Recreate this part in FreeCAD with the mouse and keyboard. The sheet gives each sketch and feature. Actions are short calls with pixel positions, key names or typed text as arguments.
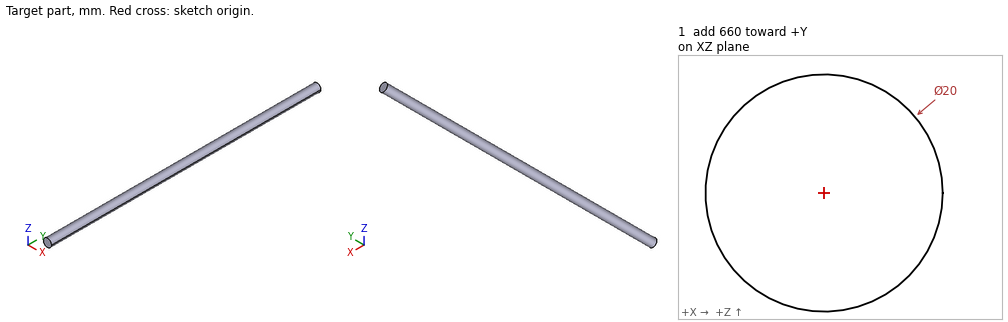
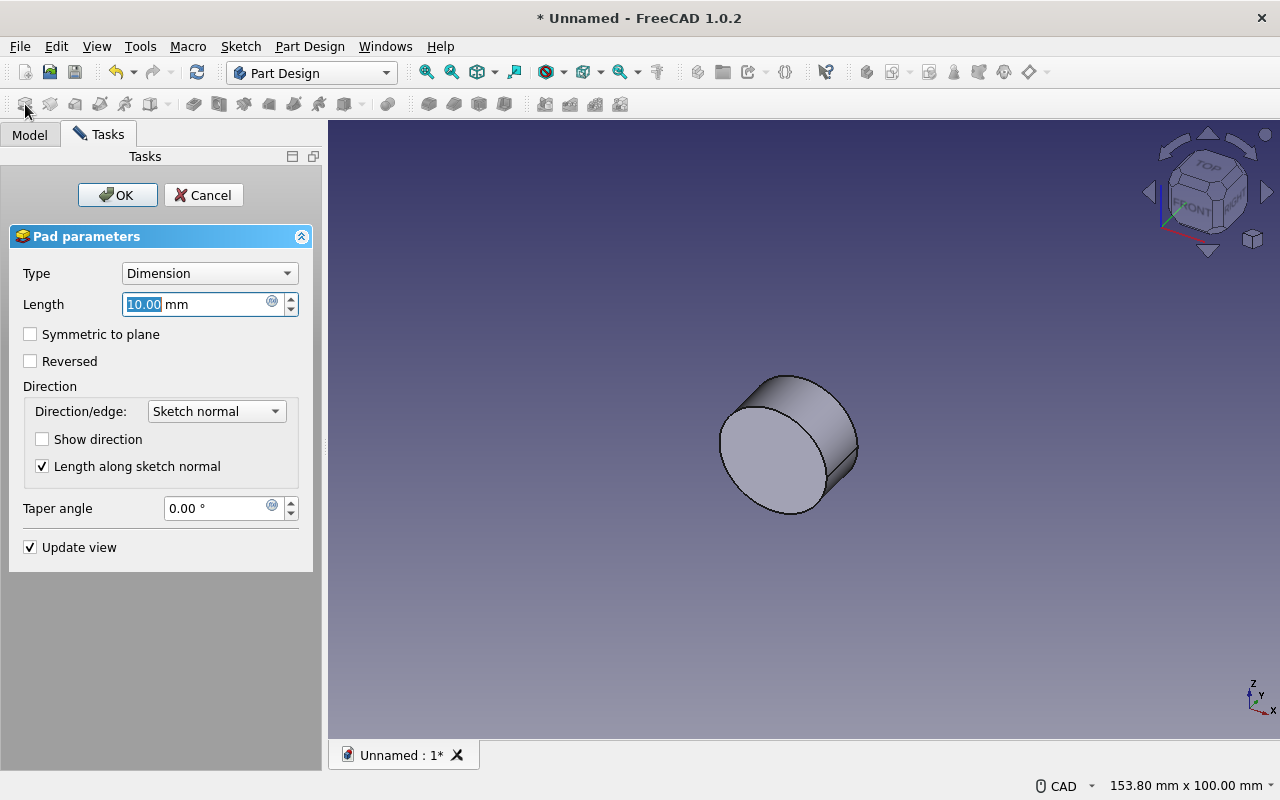
text(660)
key(Tab)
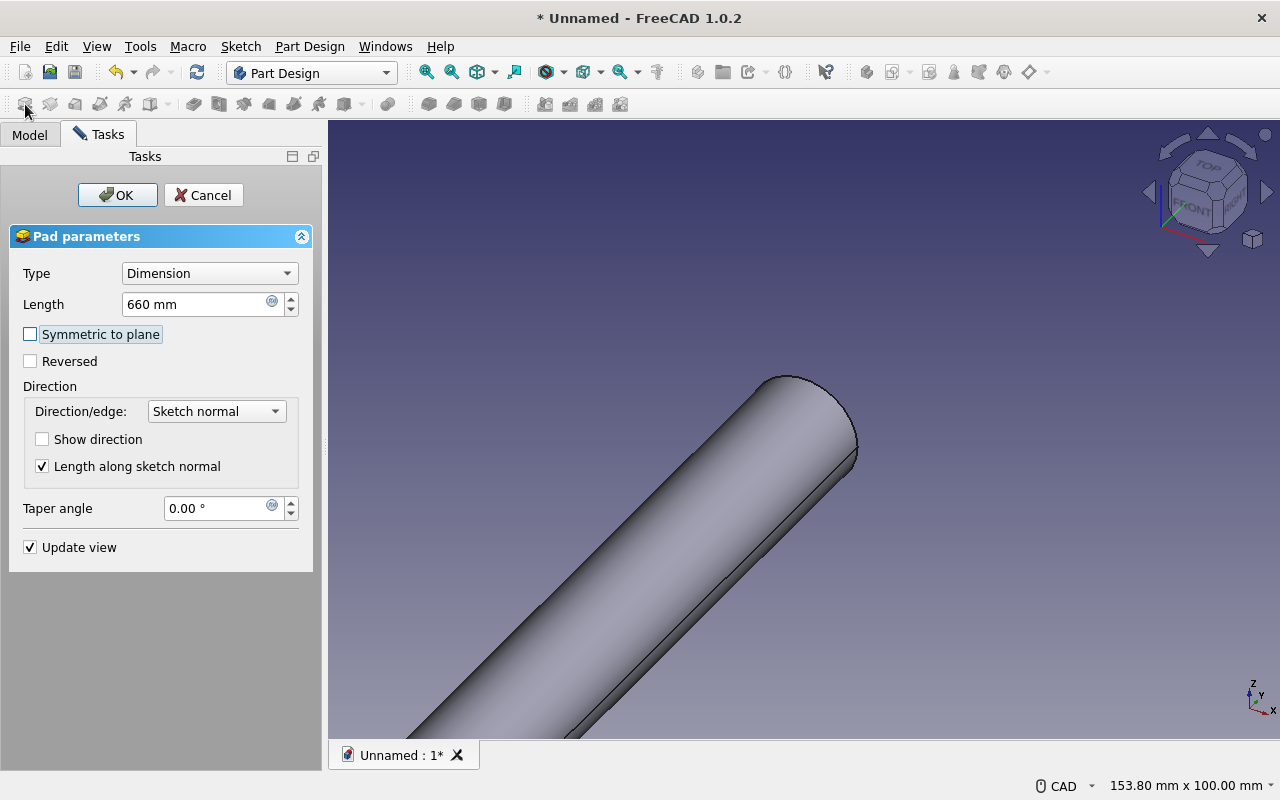
click(31, 361)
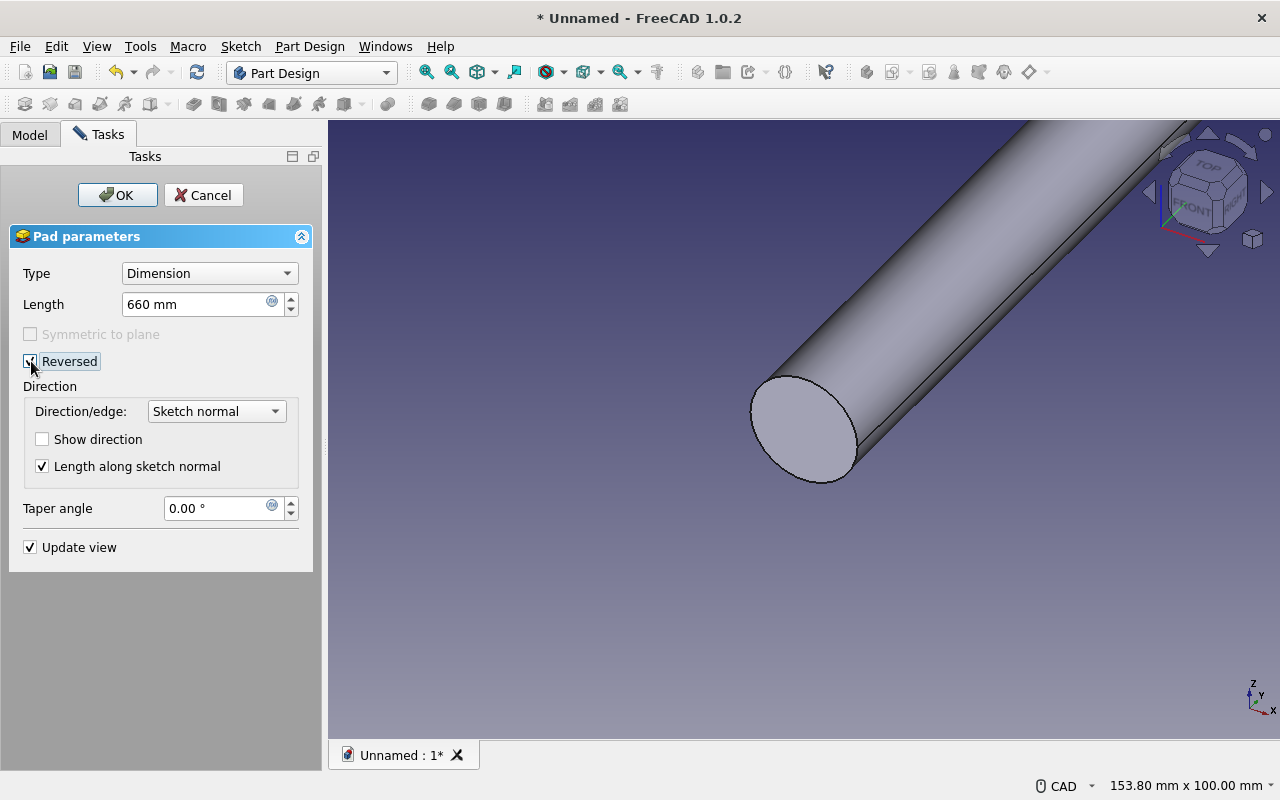
click(118, 195)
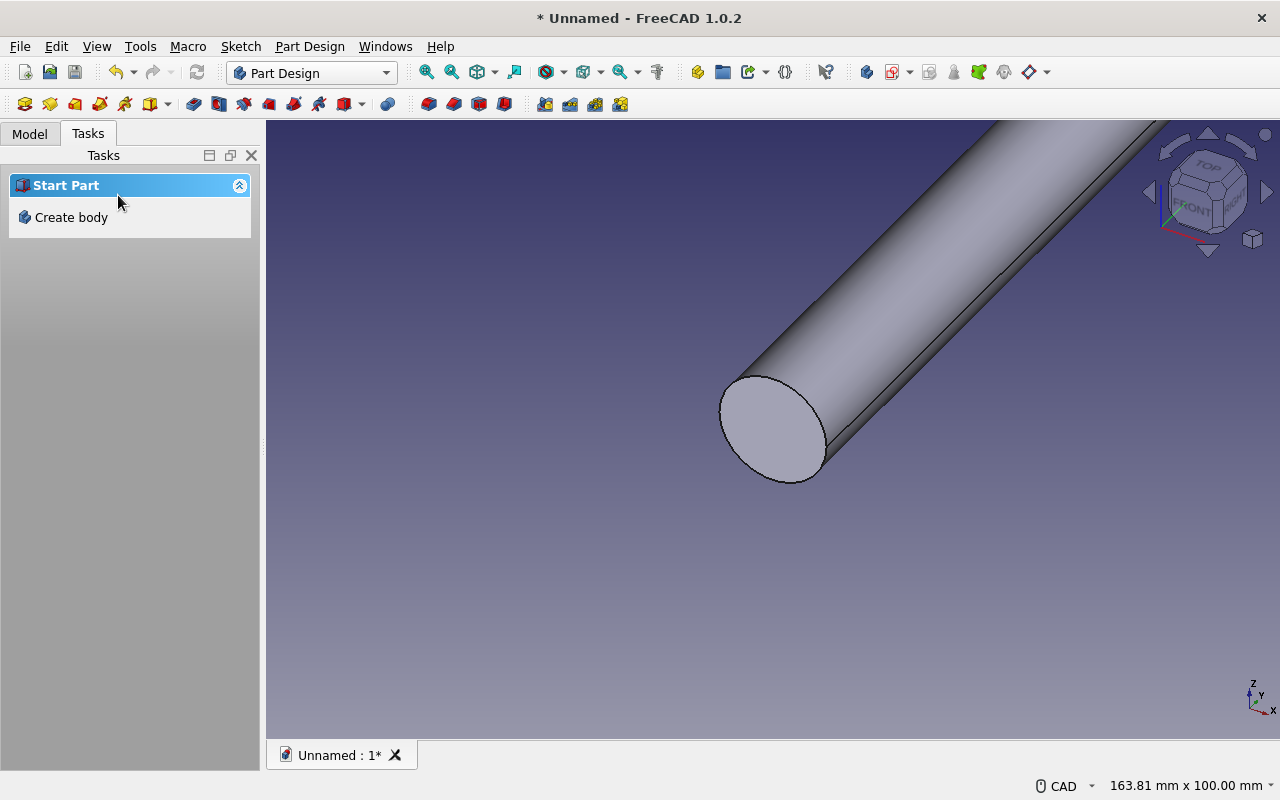
key(0)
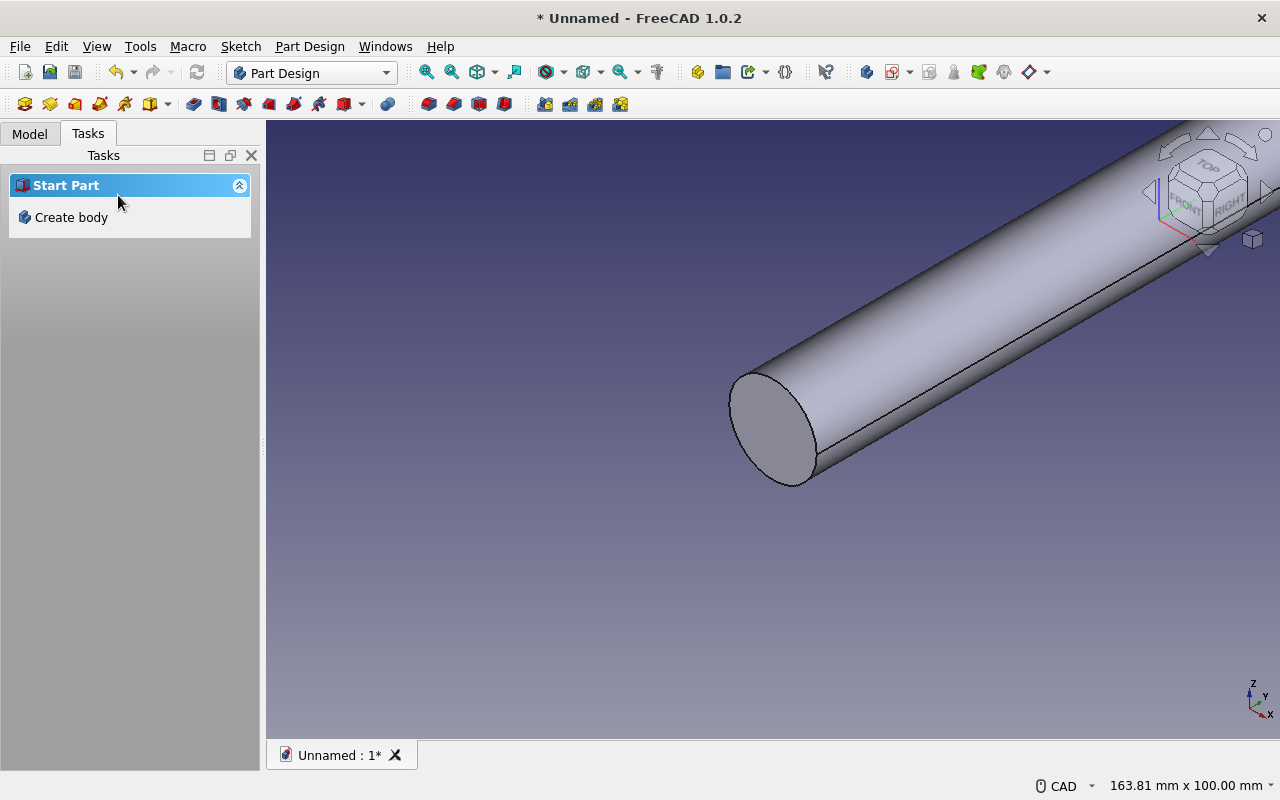
key(v)
key(f)